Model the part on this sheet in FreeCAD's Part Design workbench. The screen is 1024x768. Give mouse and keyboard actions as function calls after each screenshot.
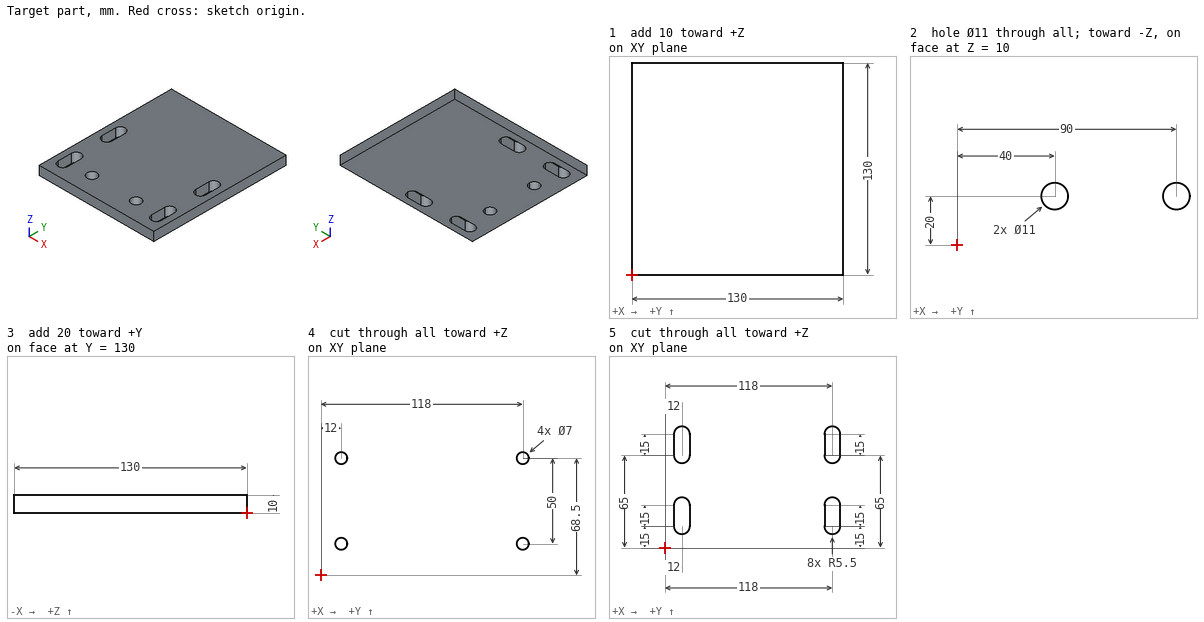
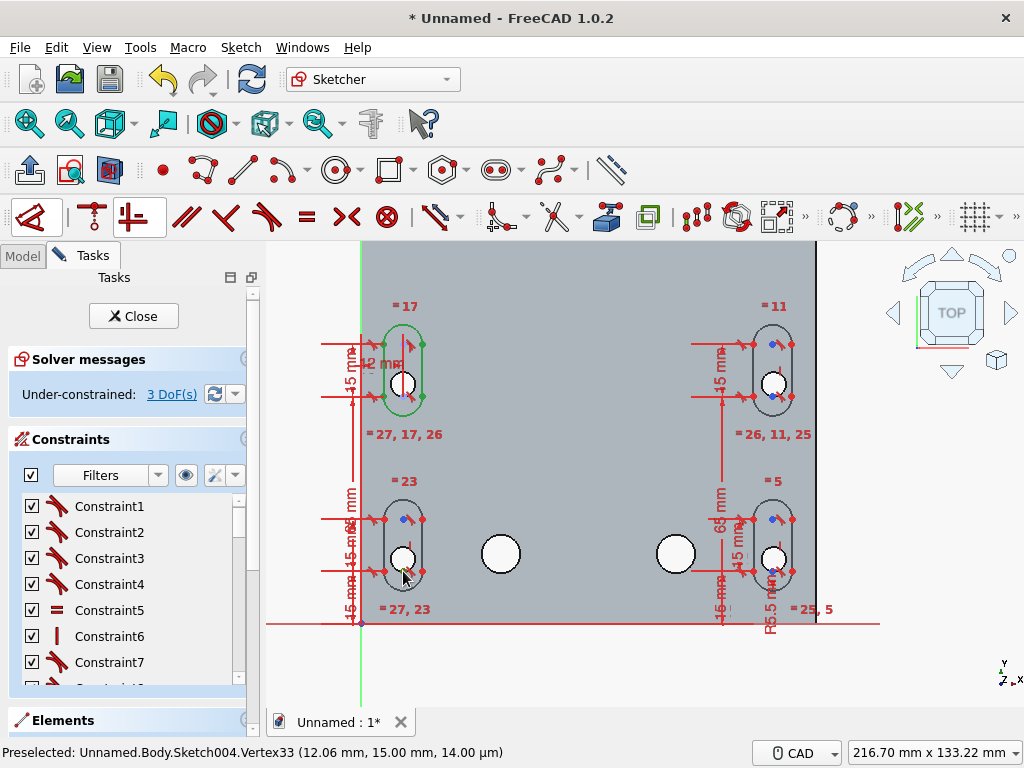
key(l)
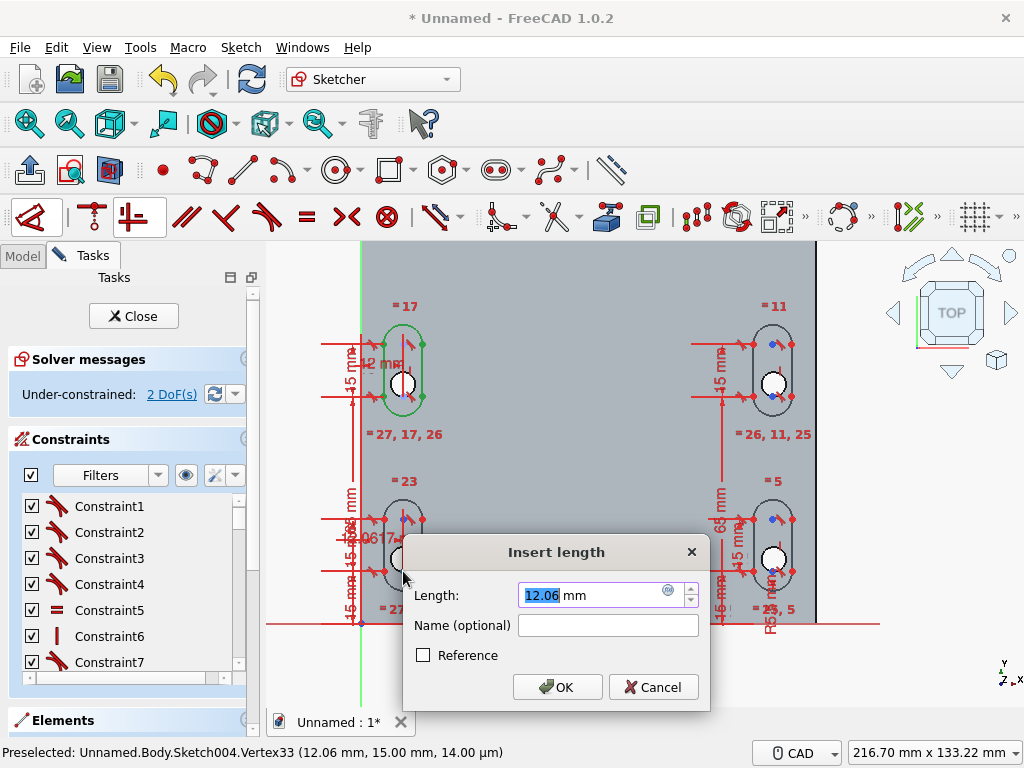
text(12)
key(Return)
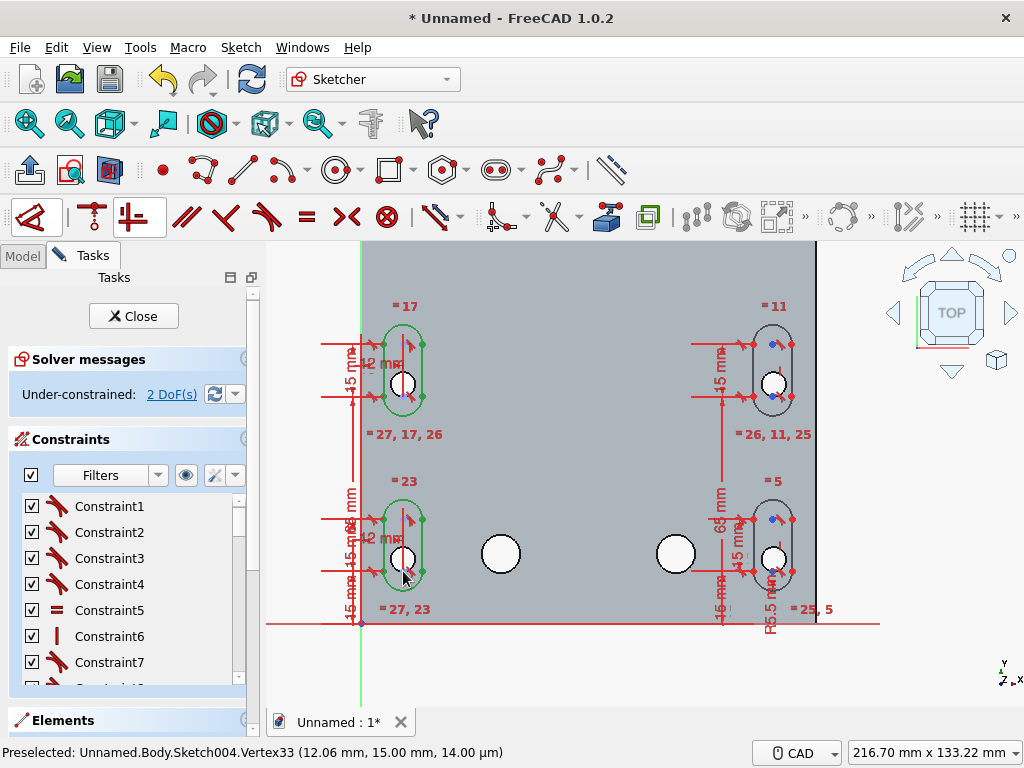
click(773, 571)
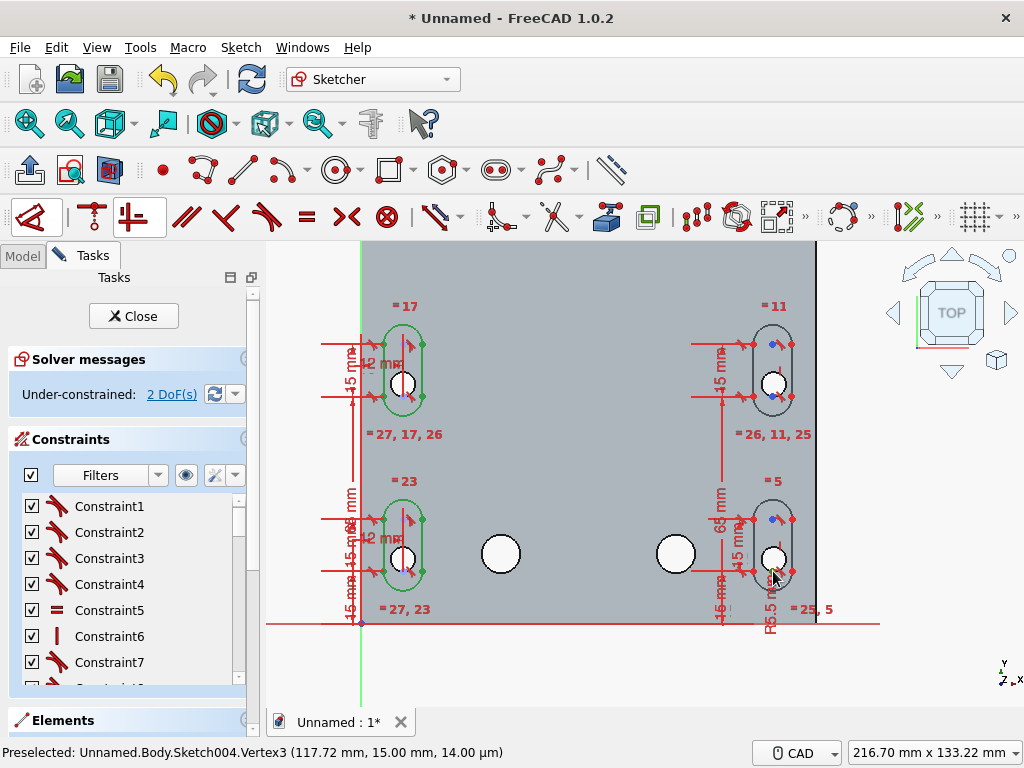
key(l)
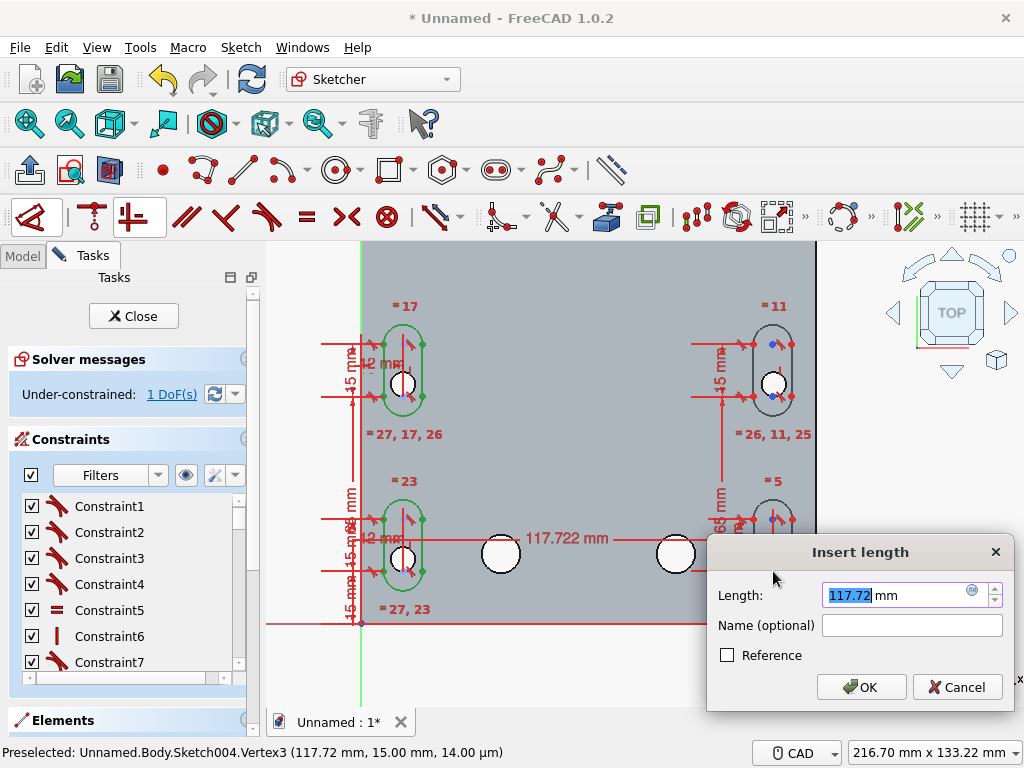
text(118)
key(Return)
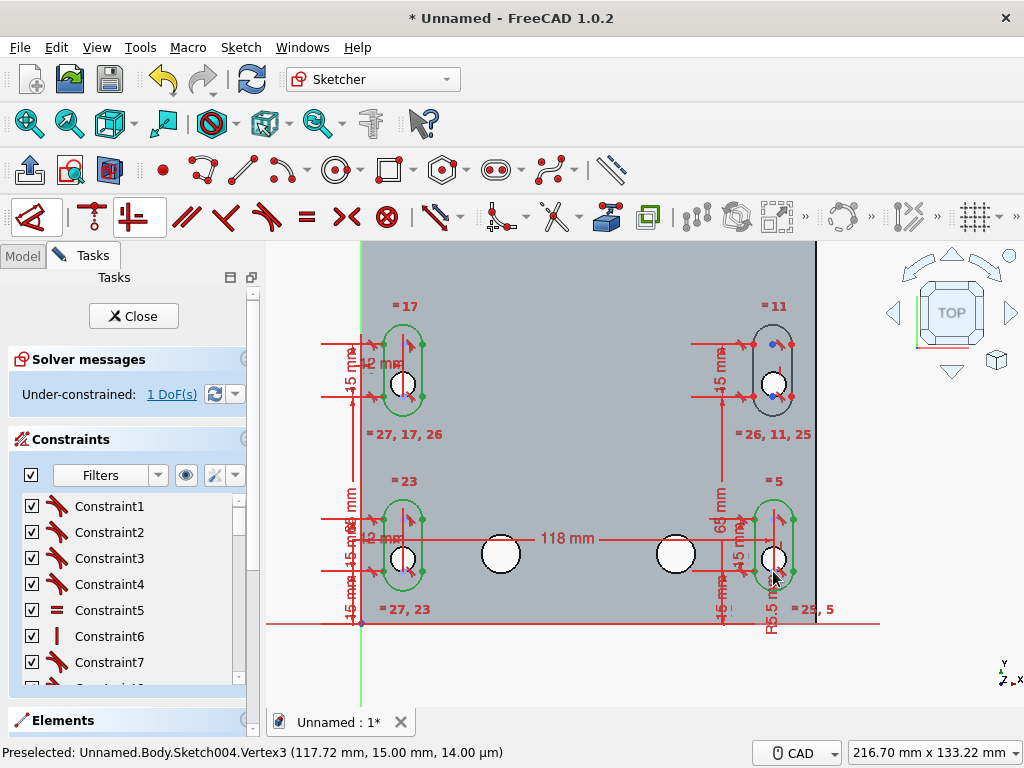
click(773, 397)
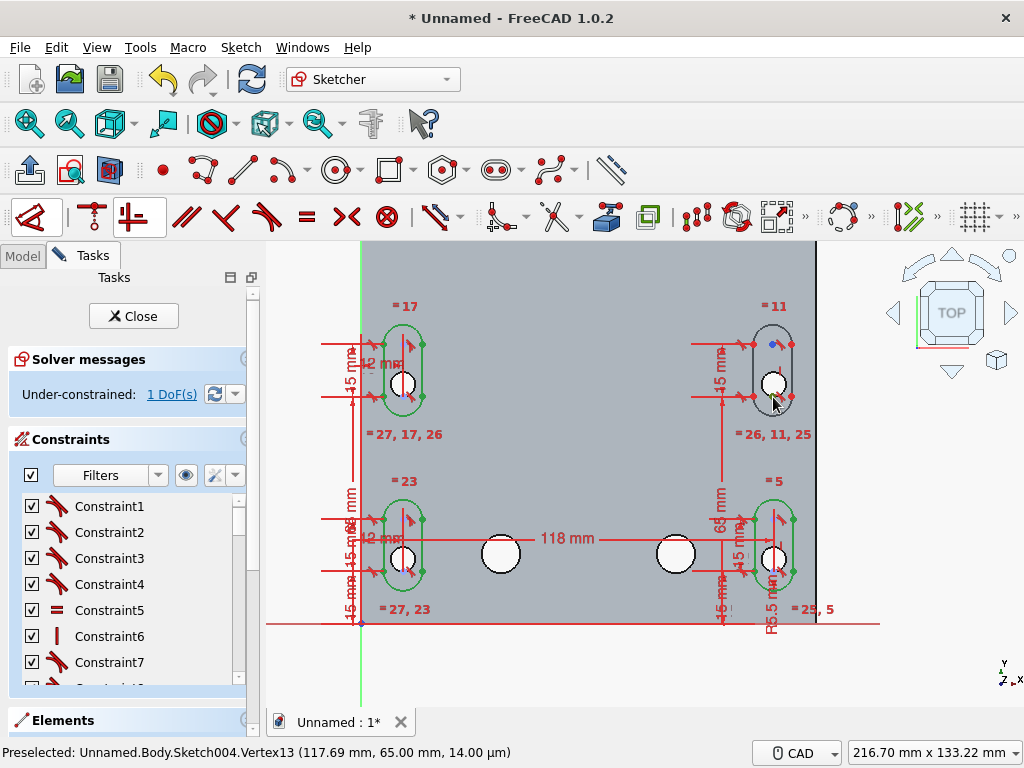
click(56, 218)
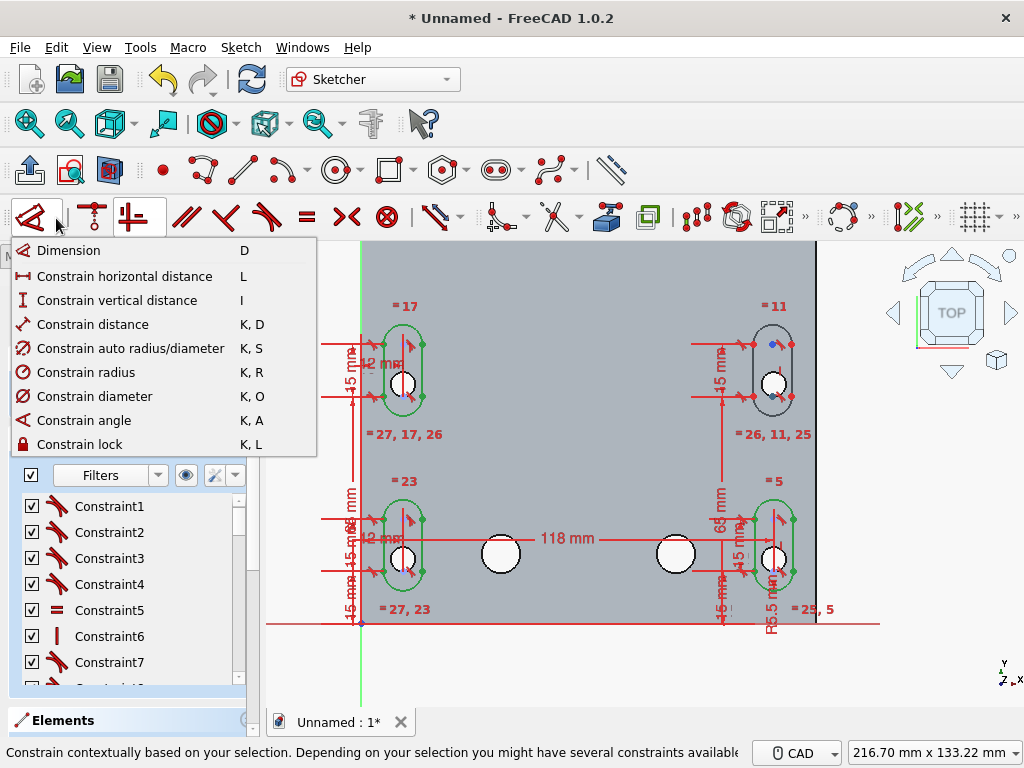
click(164, 276)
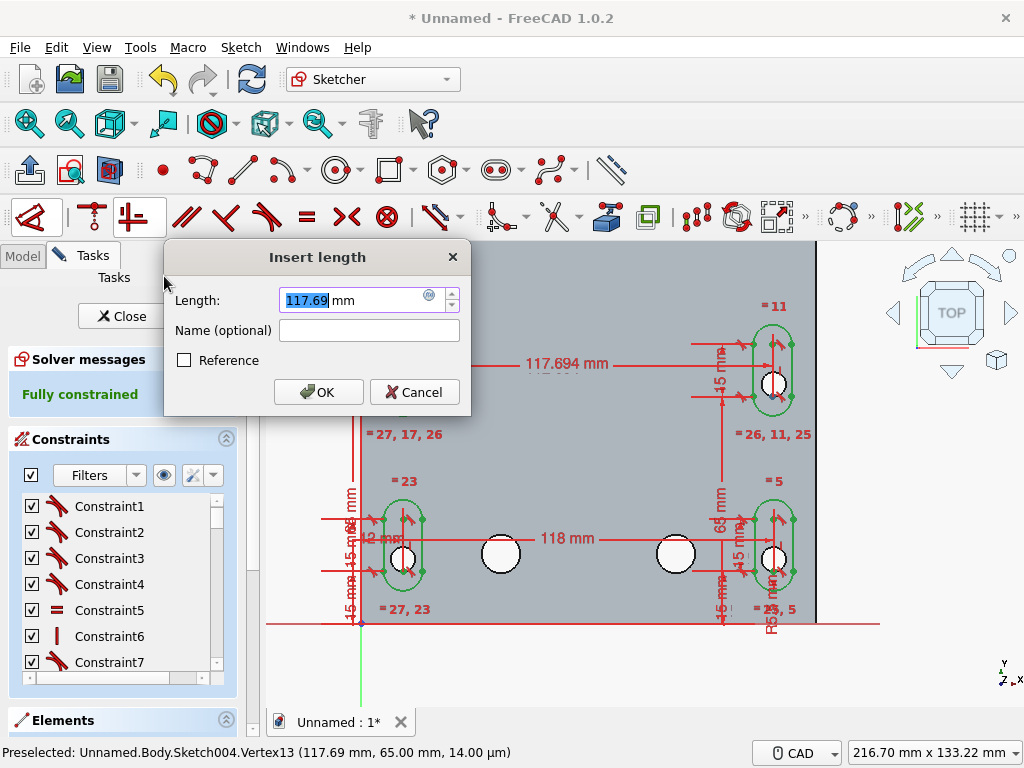
text(118)
key(Return)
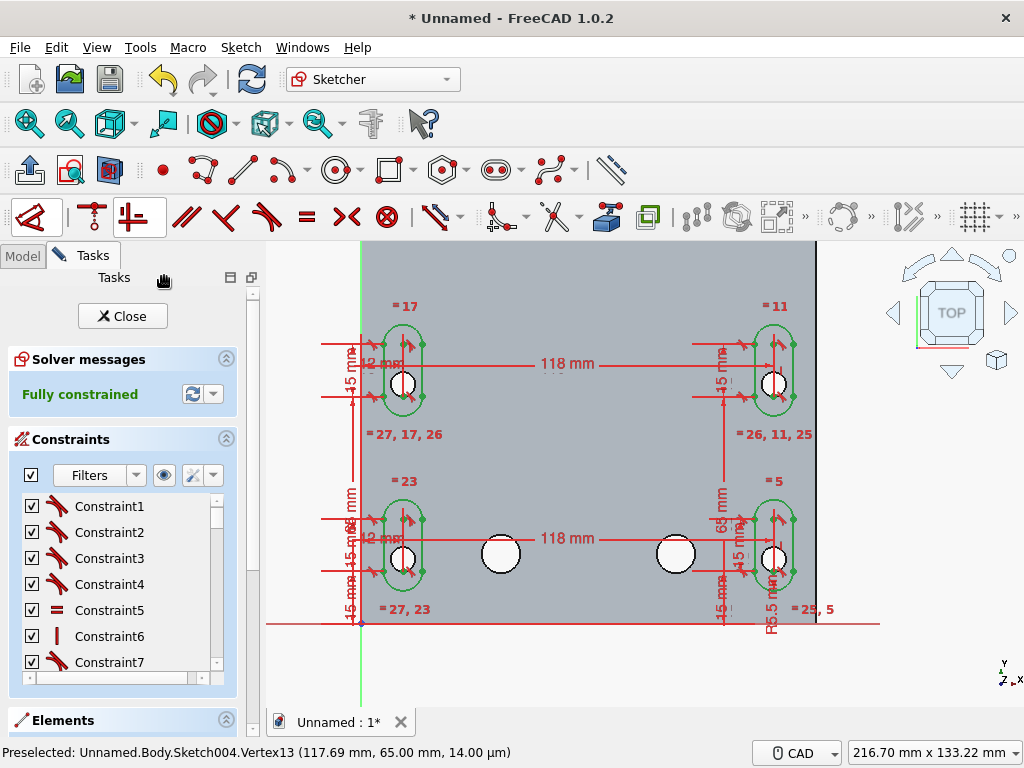
click(123, 316)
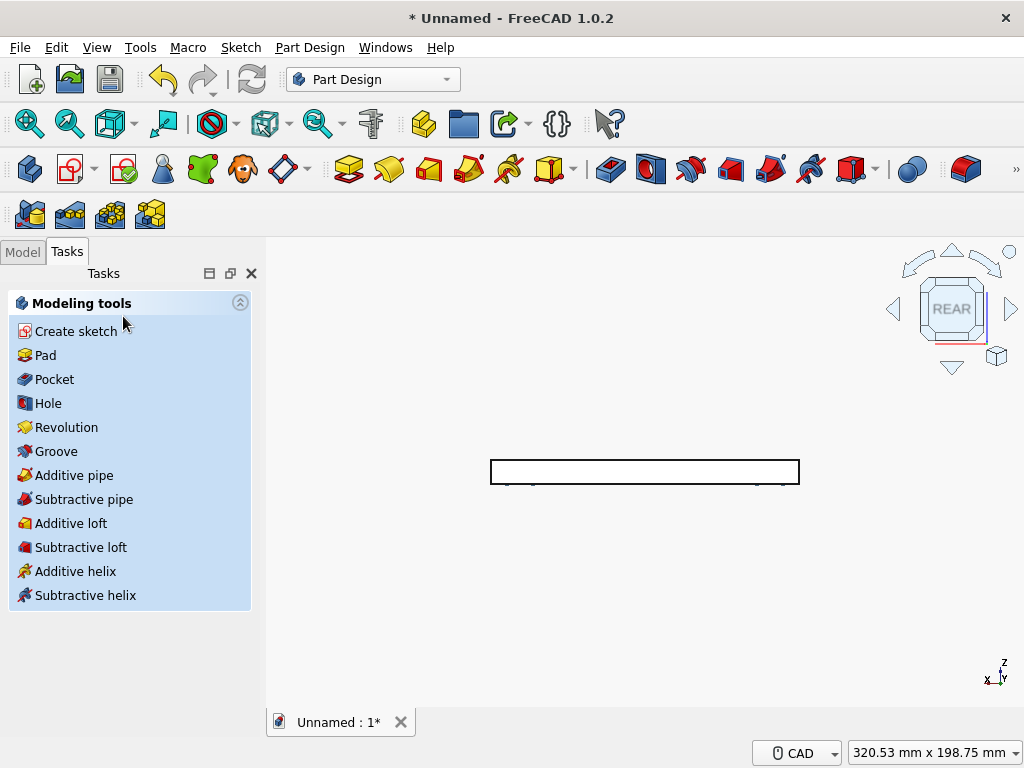
click(612, 170)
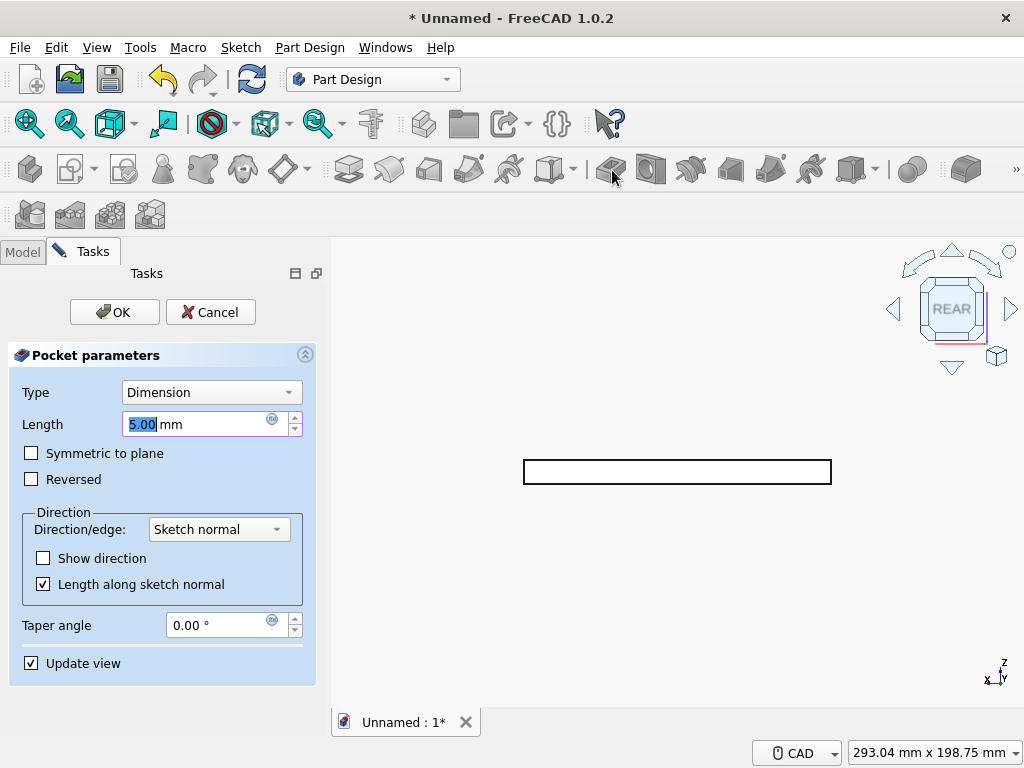
click(212, 392)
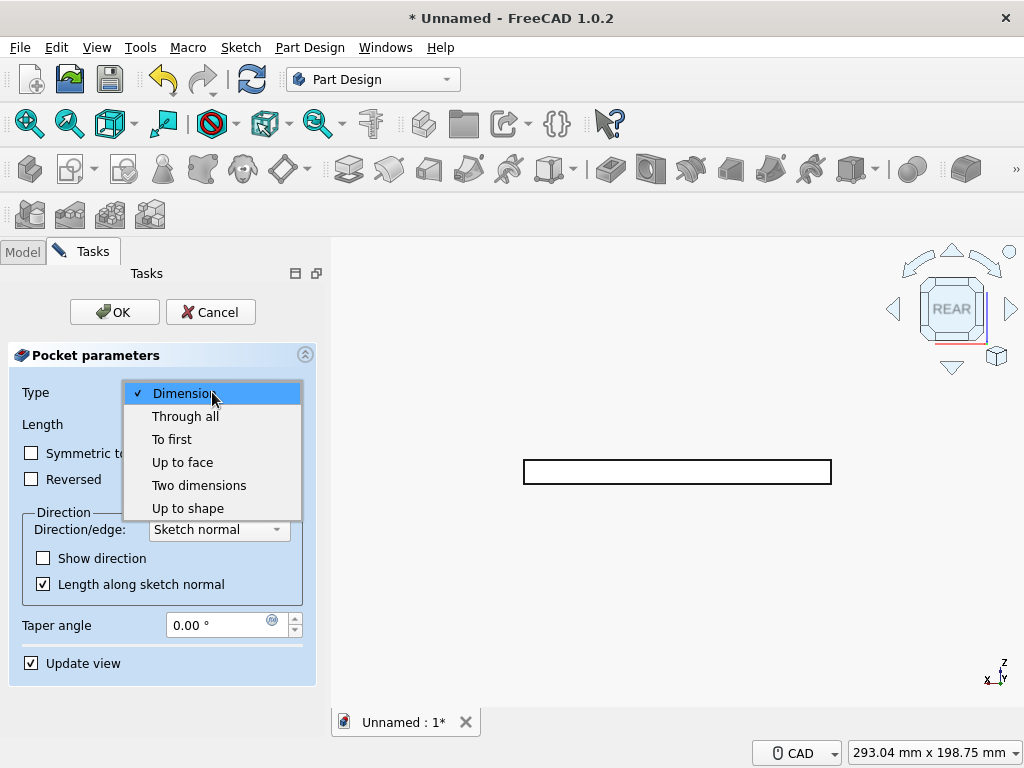
click(212, 416)